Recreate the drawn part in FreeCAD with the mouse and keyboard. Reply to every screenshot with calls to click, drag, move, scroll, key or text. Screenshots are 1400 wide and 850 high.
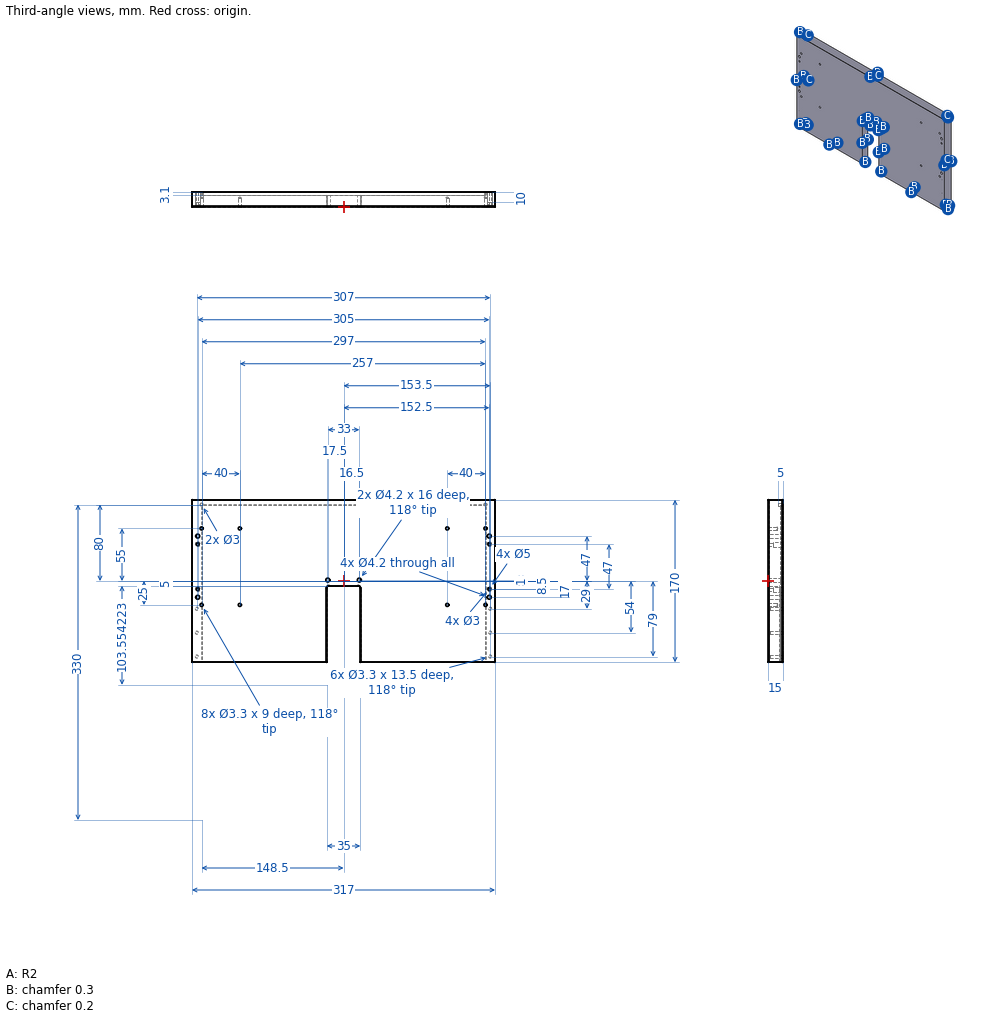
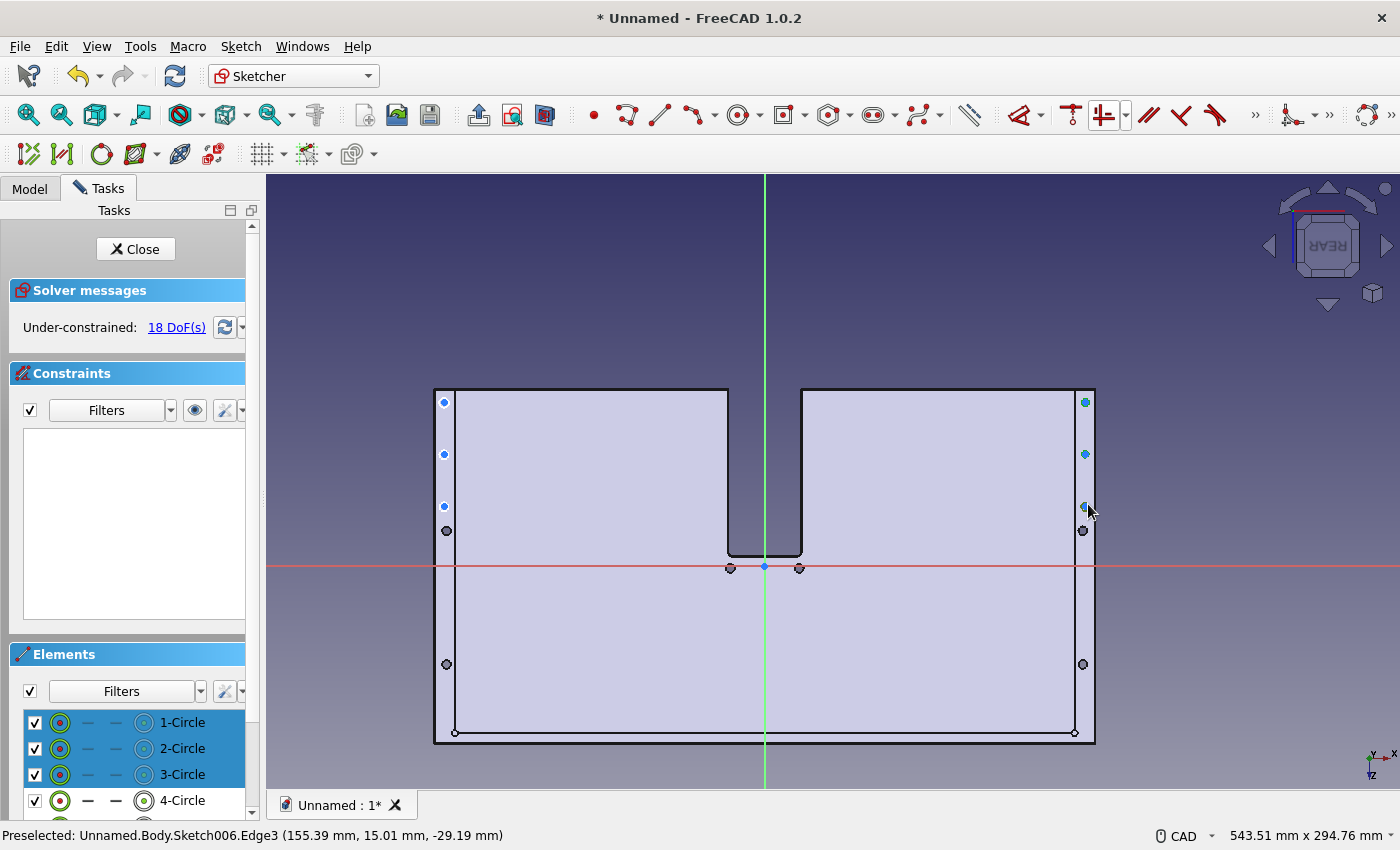
scroll(447, 504, up, 6)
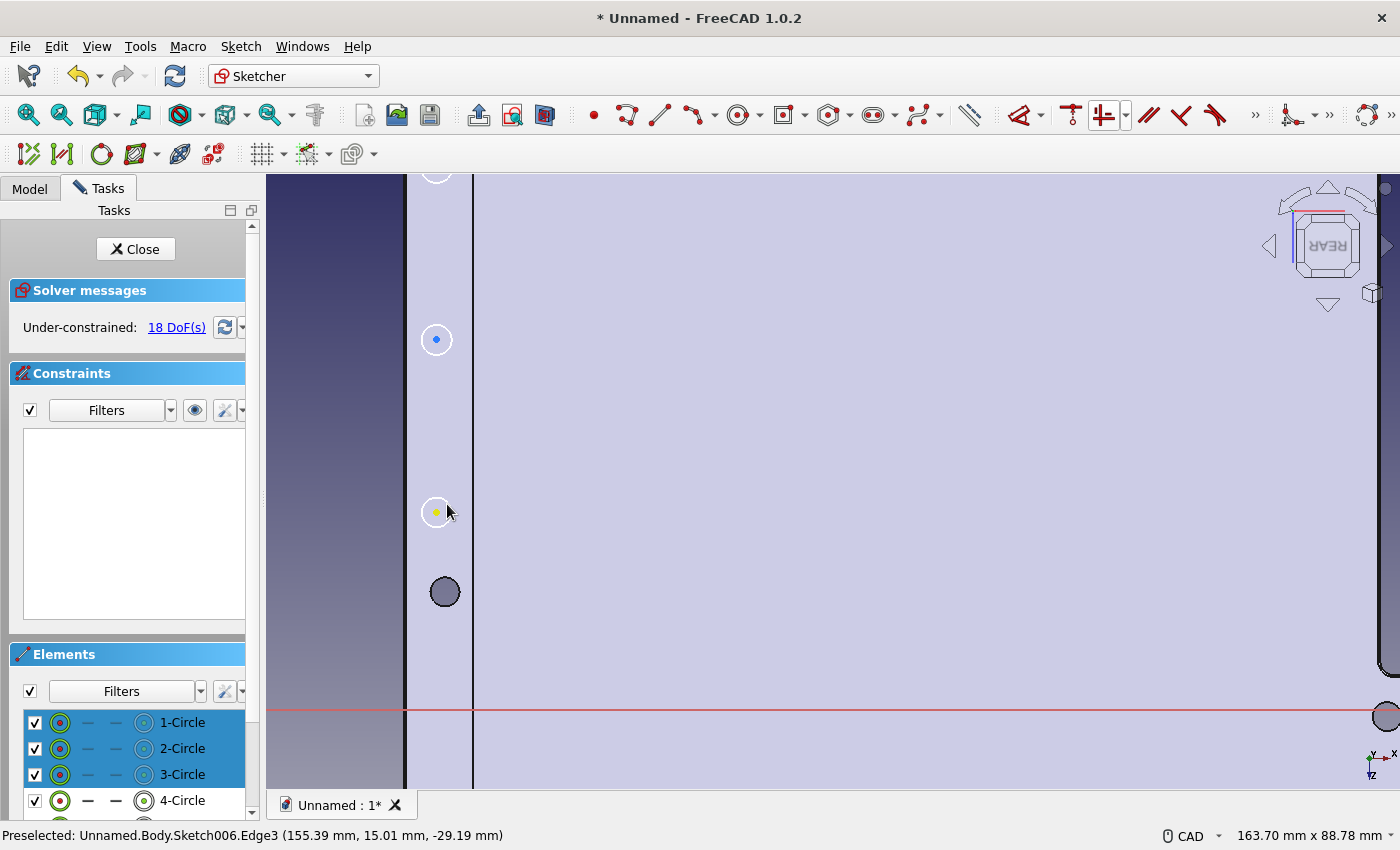
click(447, 502)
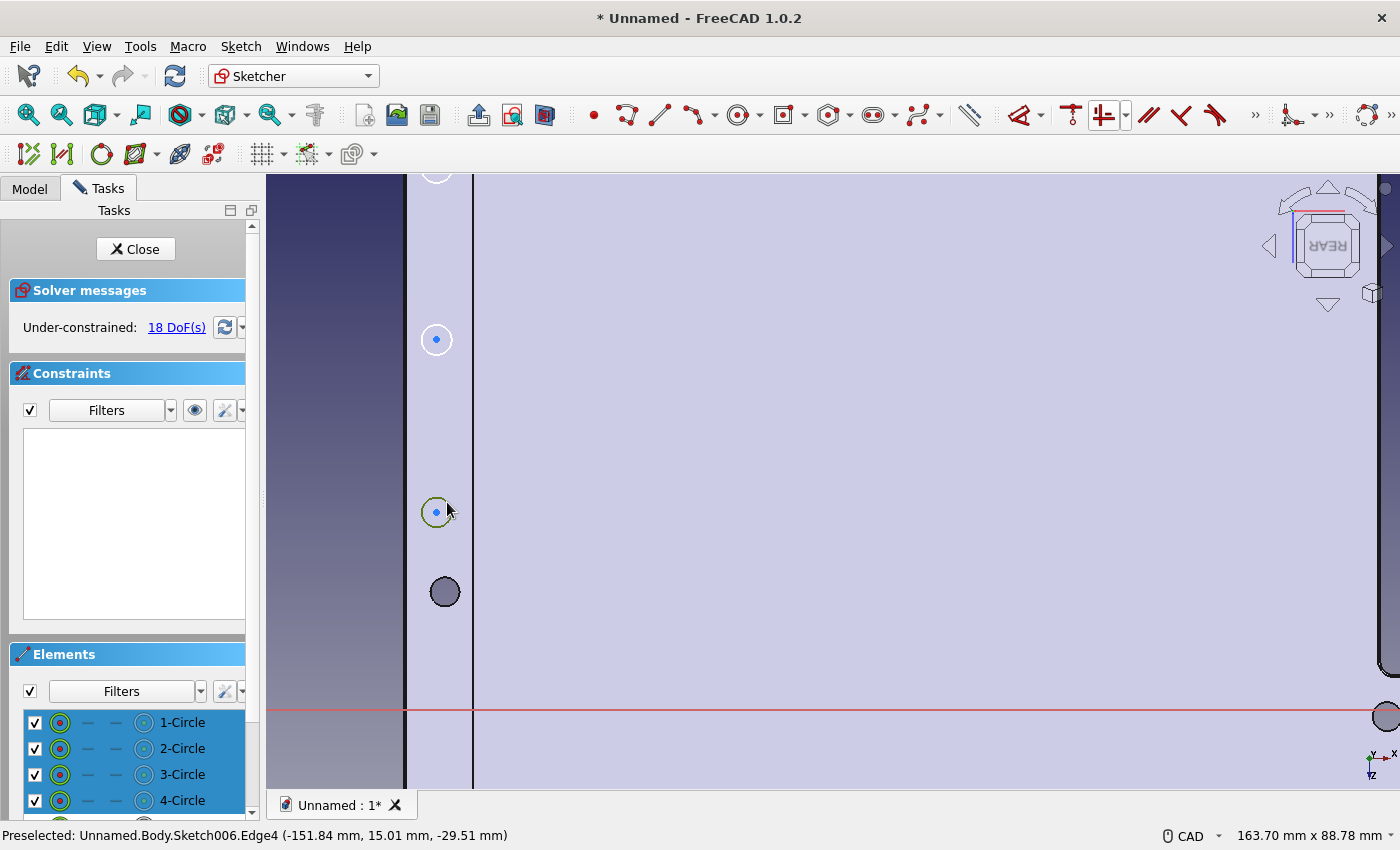
click(447, 329)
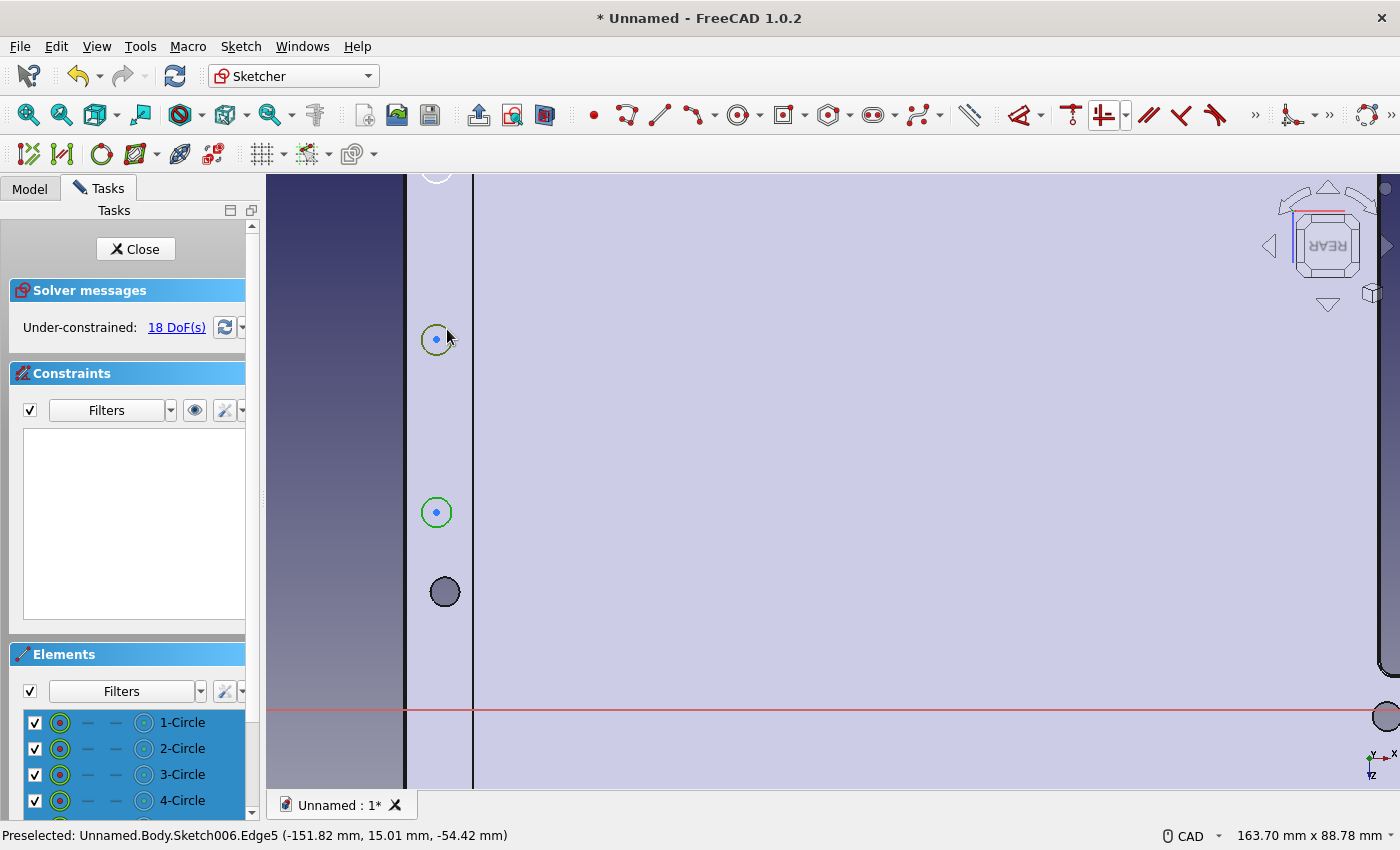
scroll(447, 504, down, 6)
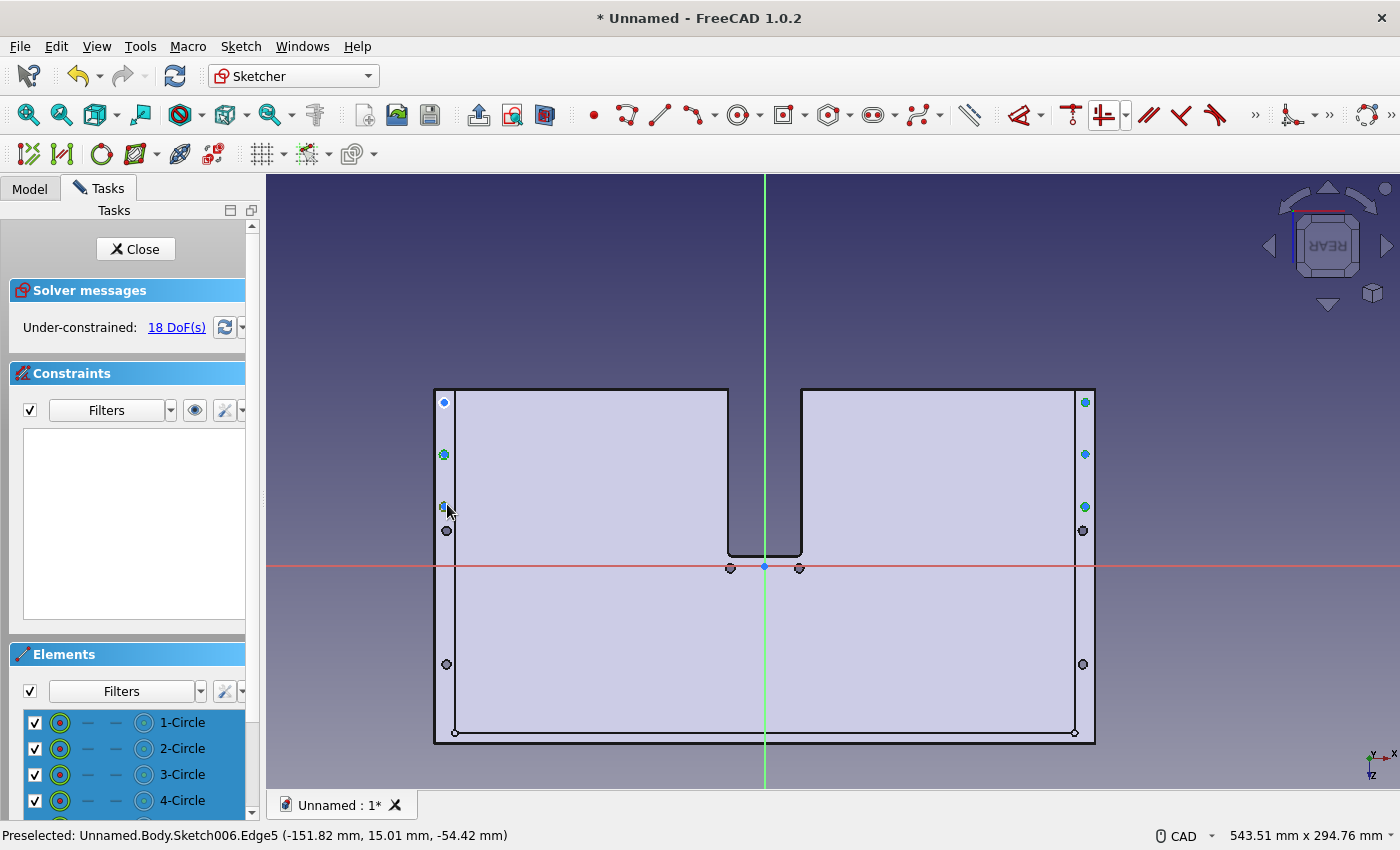
scroll(447, 400, up, 6)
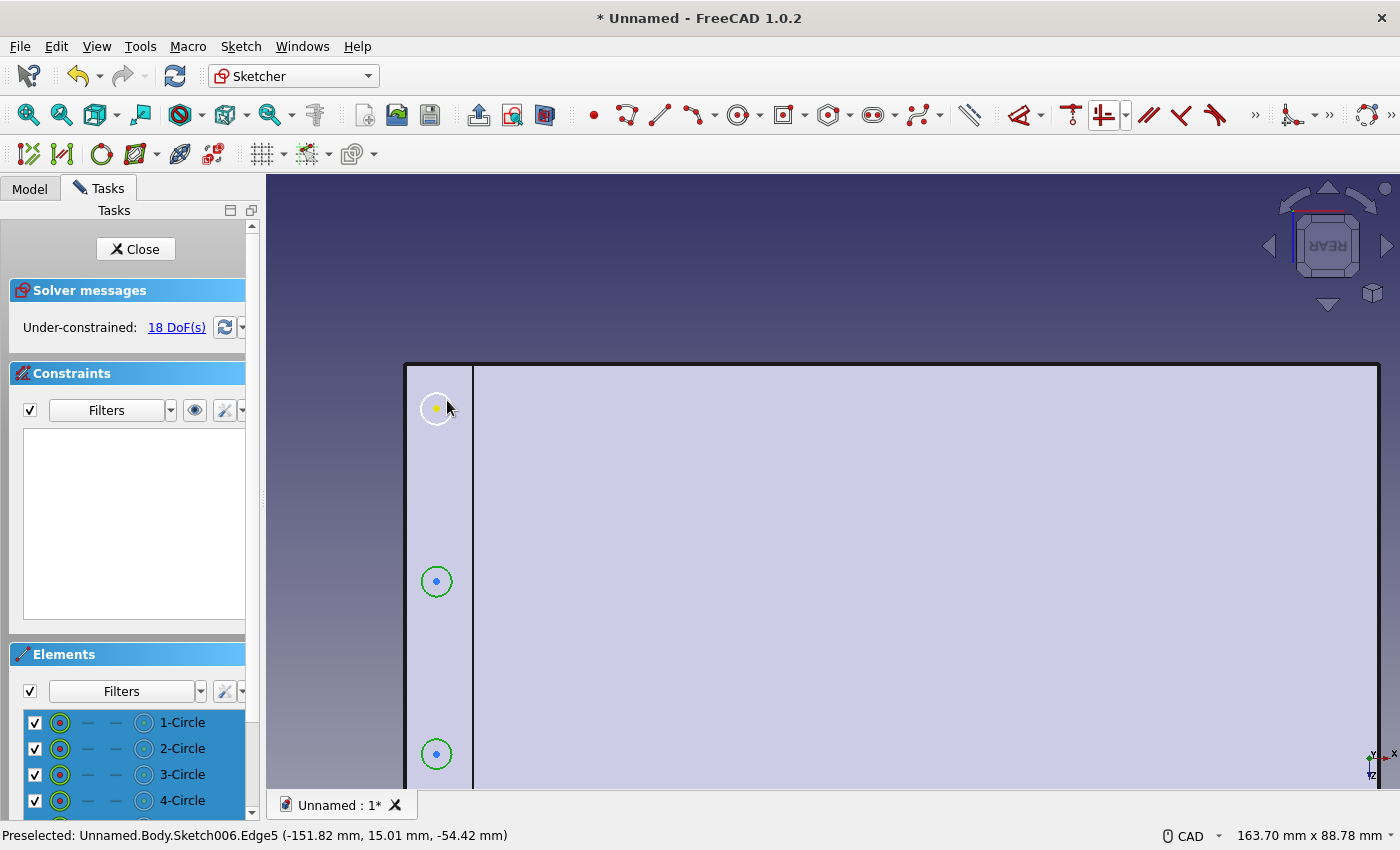
click(448, 398)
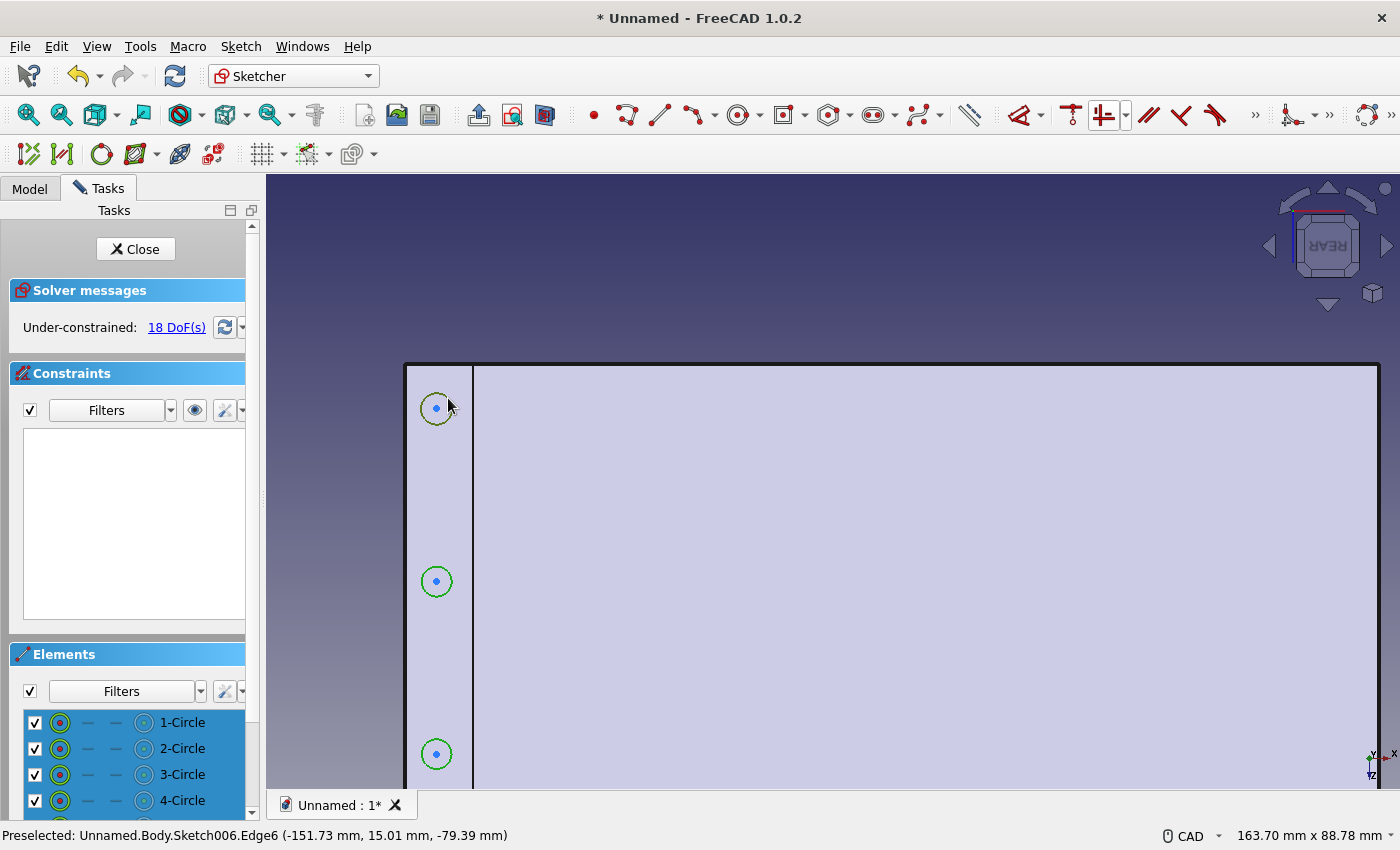
key(e)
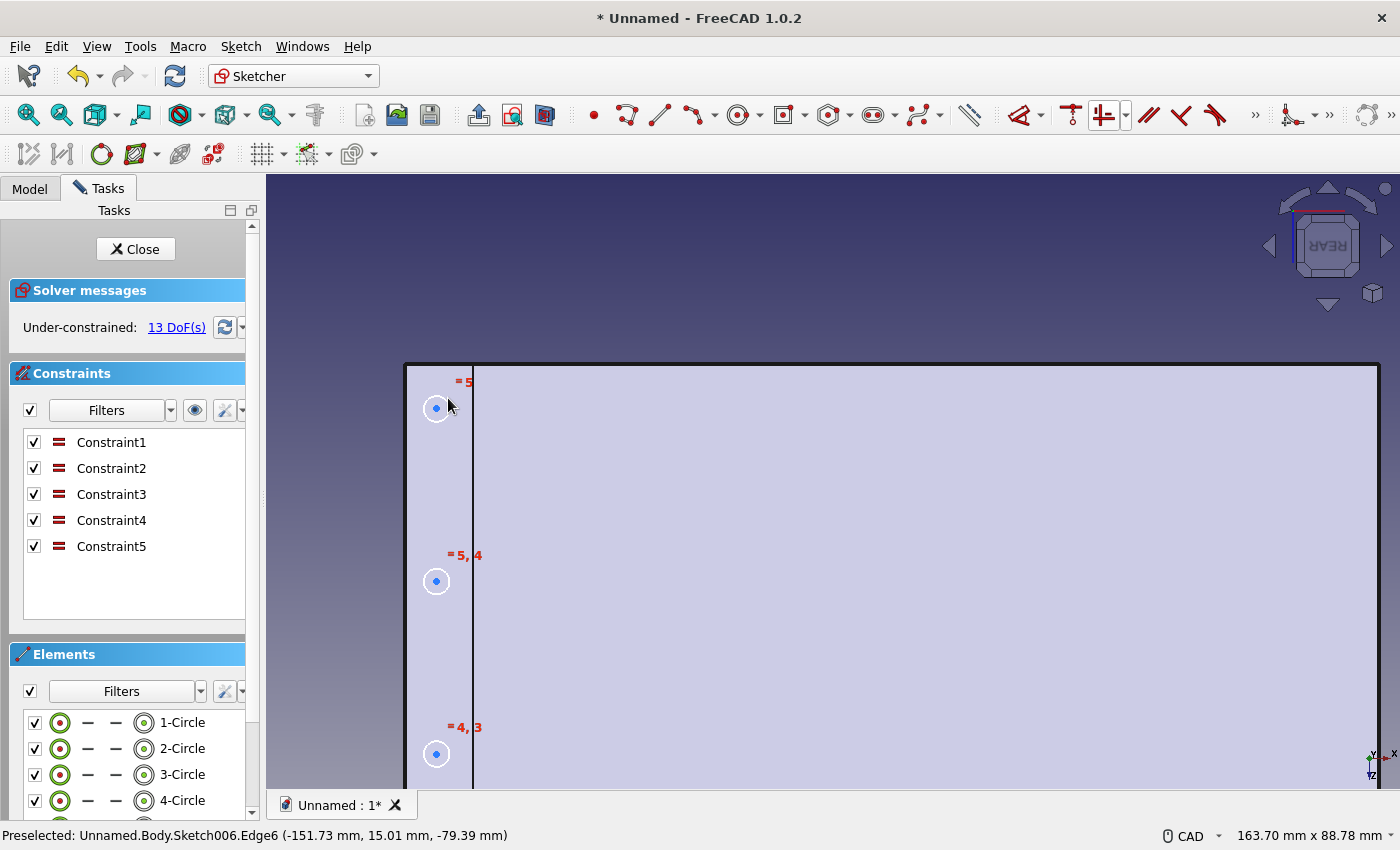
scroll(447, 399, down, 6)